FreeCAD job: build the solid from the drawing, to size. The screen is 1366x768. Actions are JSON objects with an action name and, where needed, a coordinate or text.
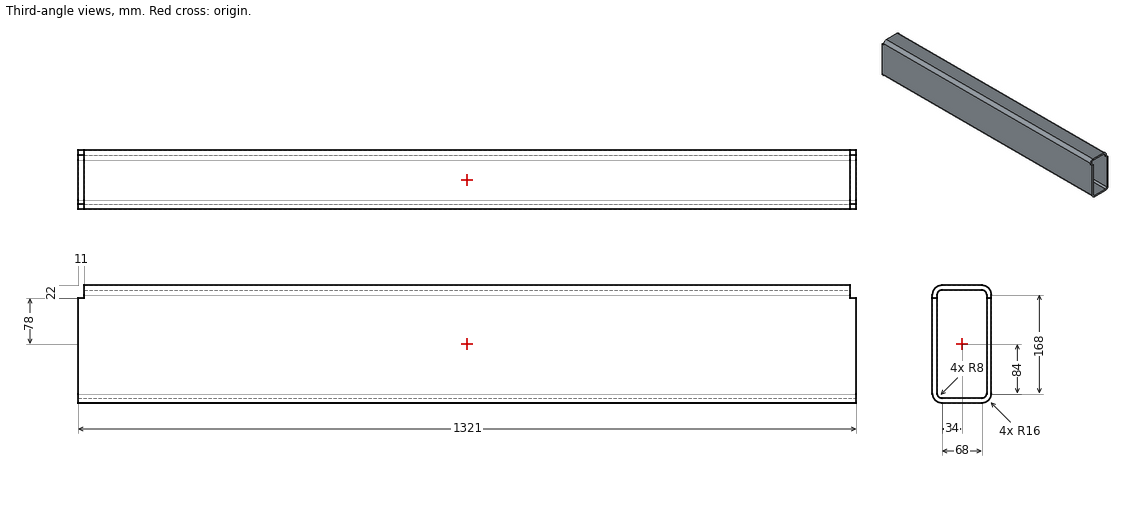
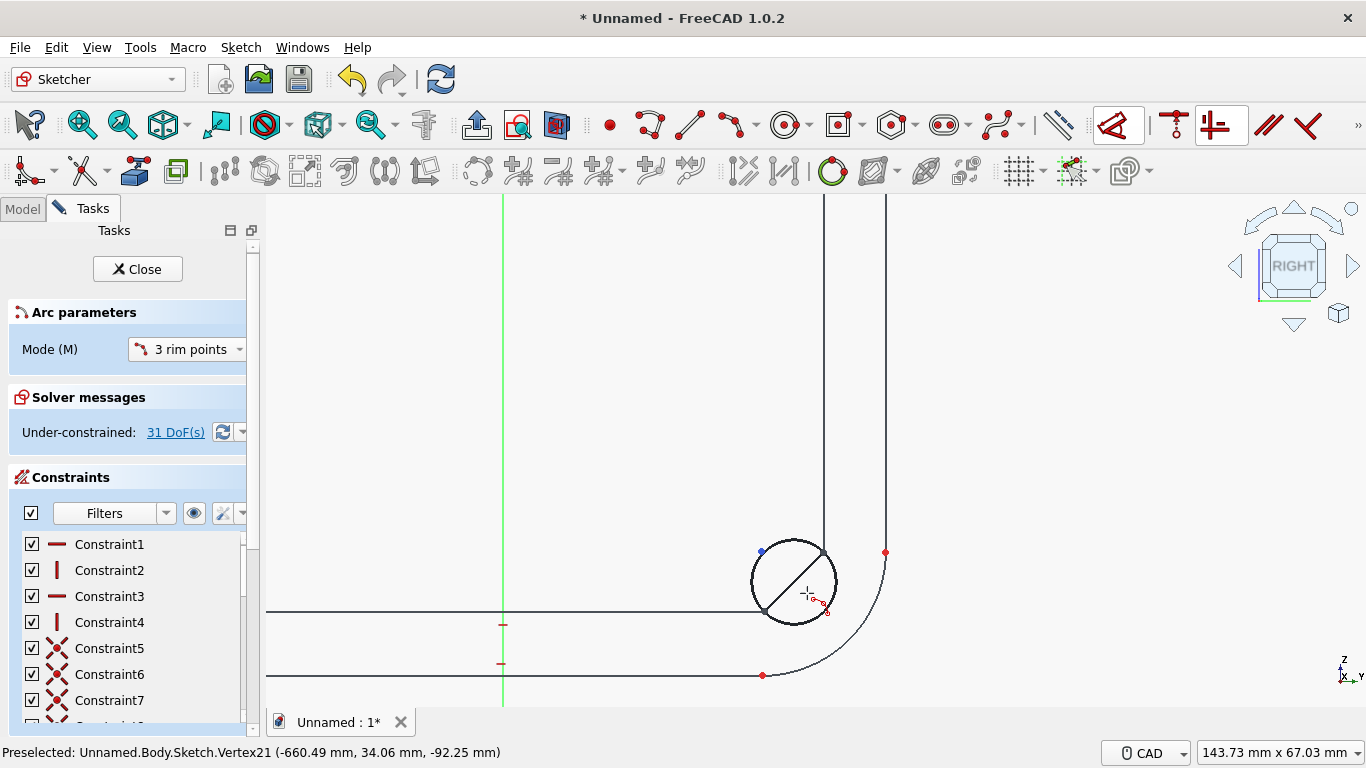
{"action": "left_click", "coordinate": [807, 592]}
{"action": "key", "text": "Escape"}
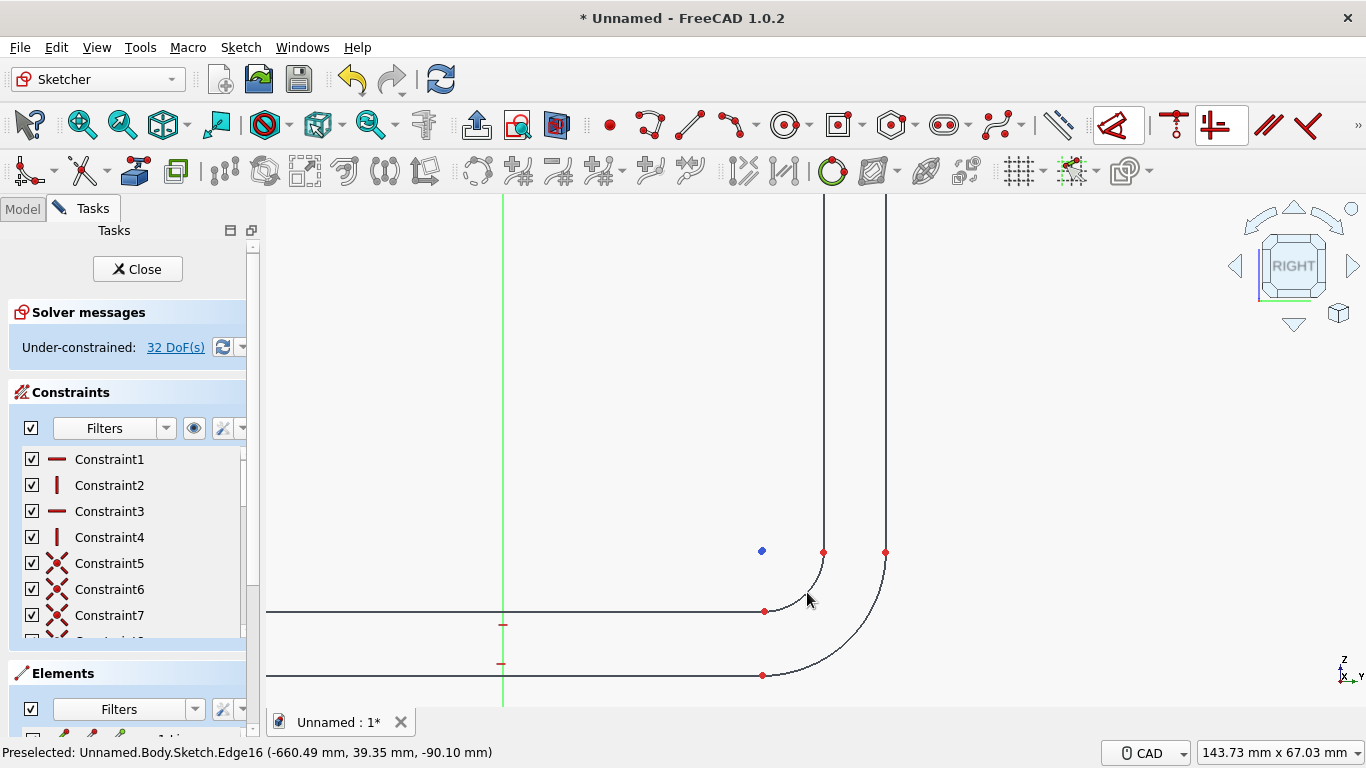
{"action": "scroll", "coordinate": [809, 588], "scroll_direction": "down", "scroll_amount": 8}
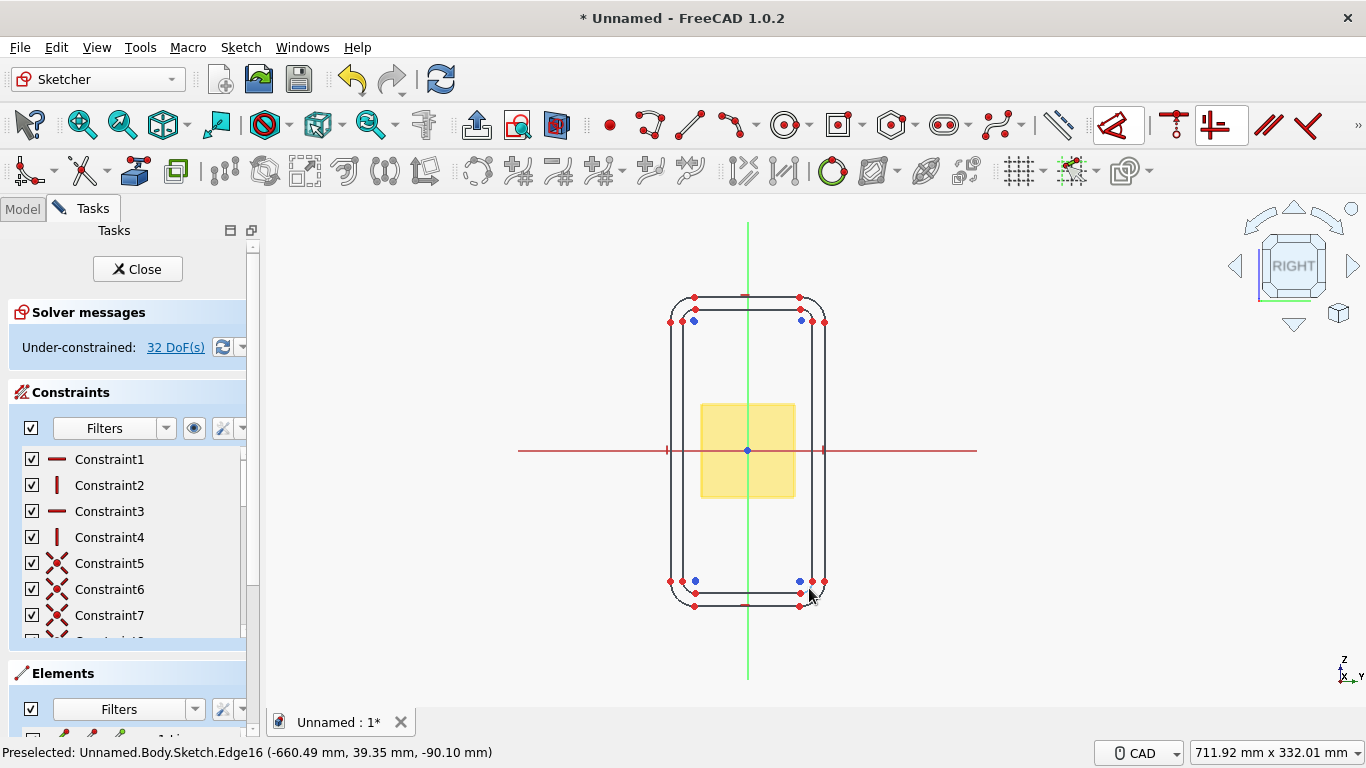
{"action": "left_click", "coordinate": [726, 606]}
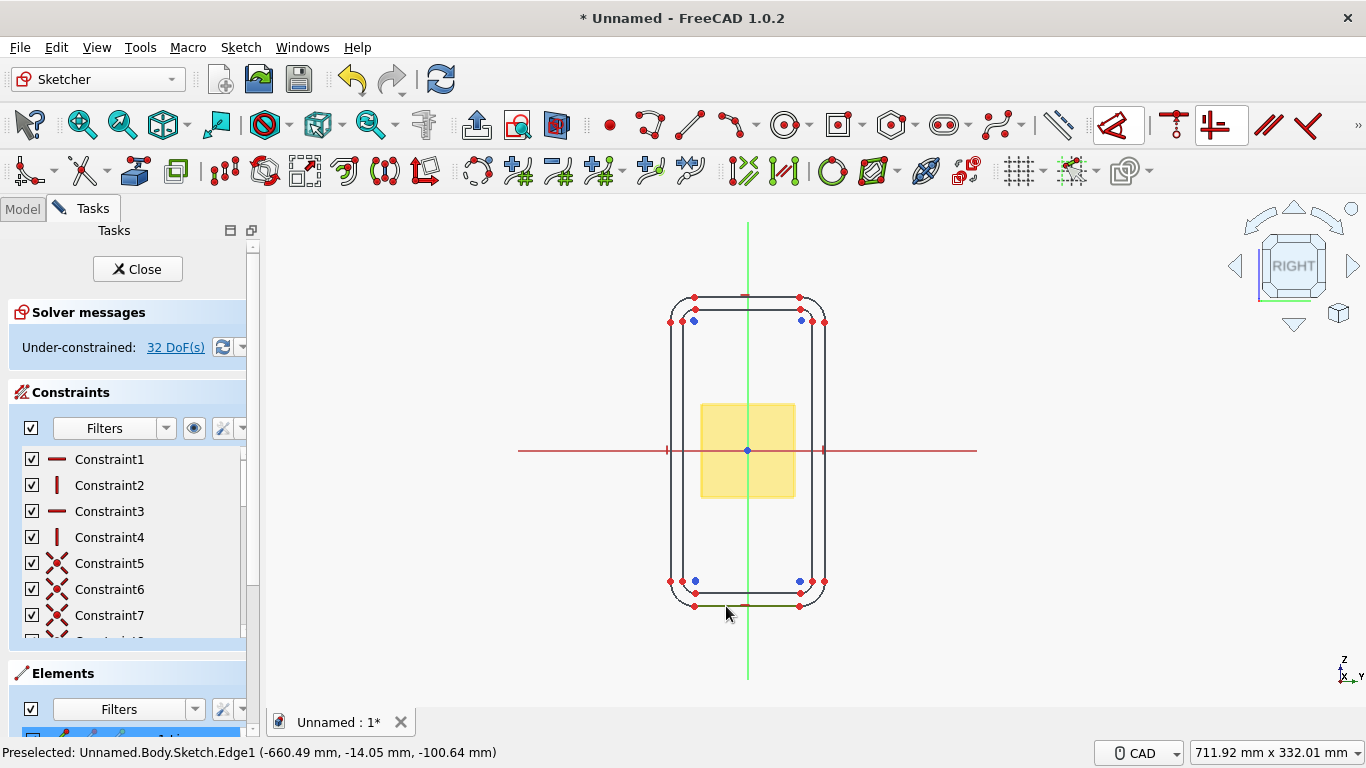
{"action": "left_click", "coordinate": [811, 604]}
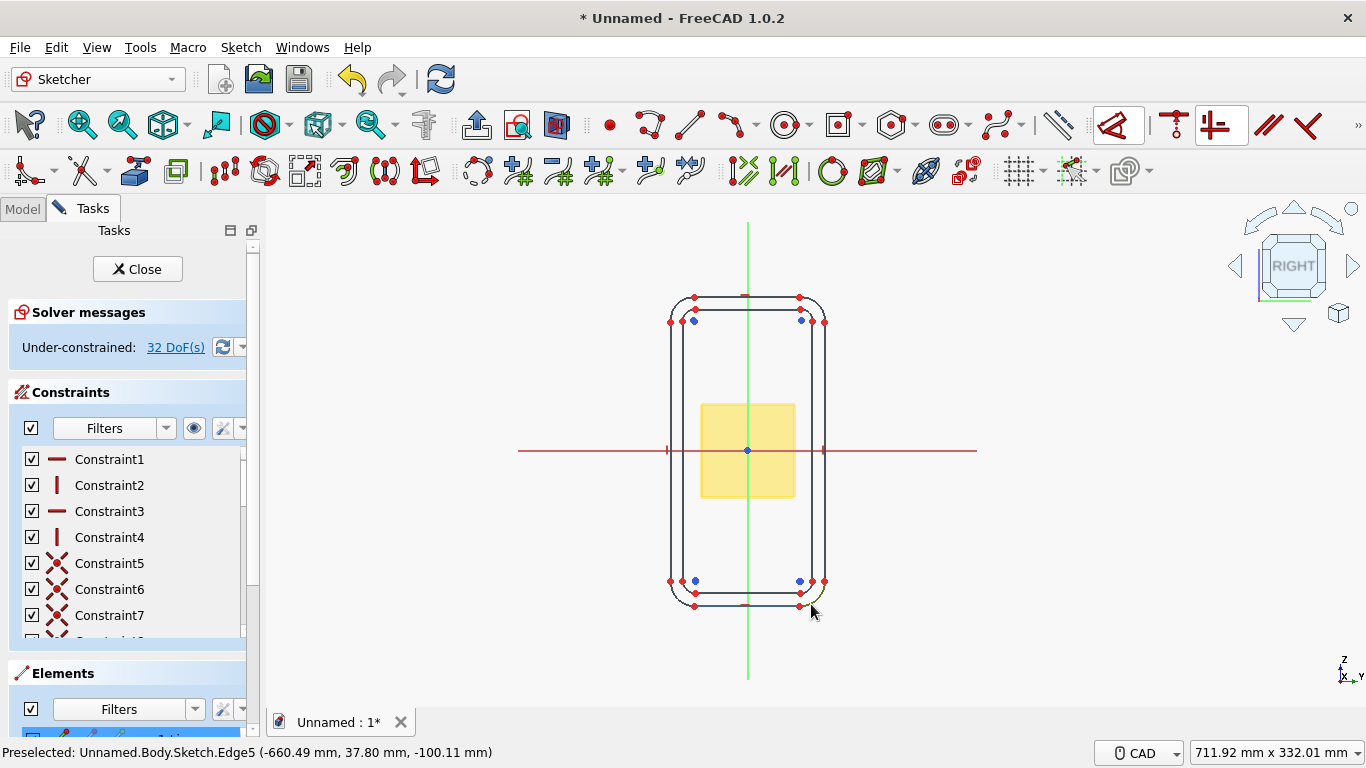
{"action": "key", "text": "t"}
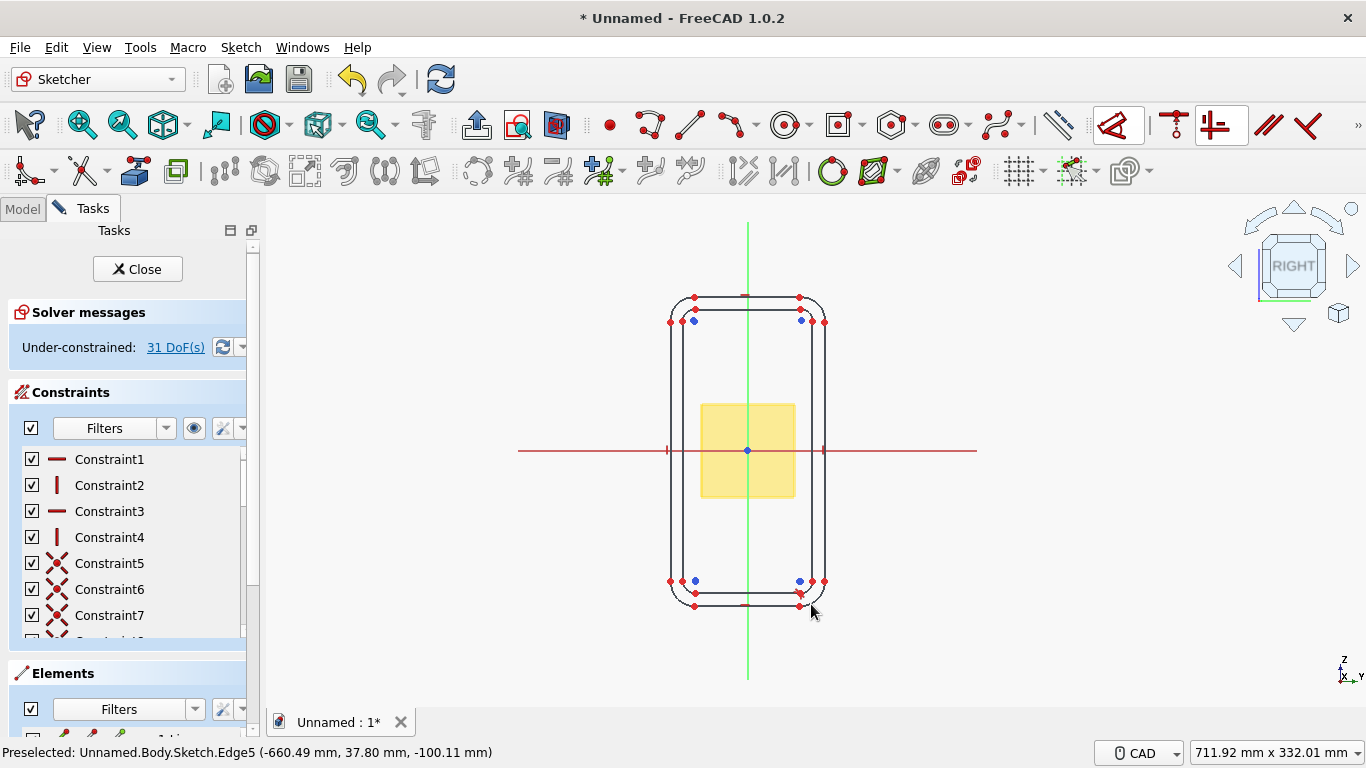
{"action": "left_click", "coordinate": [726, 606]}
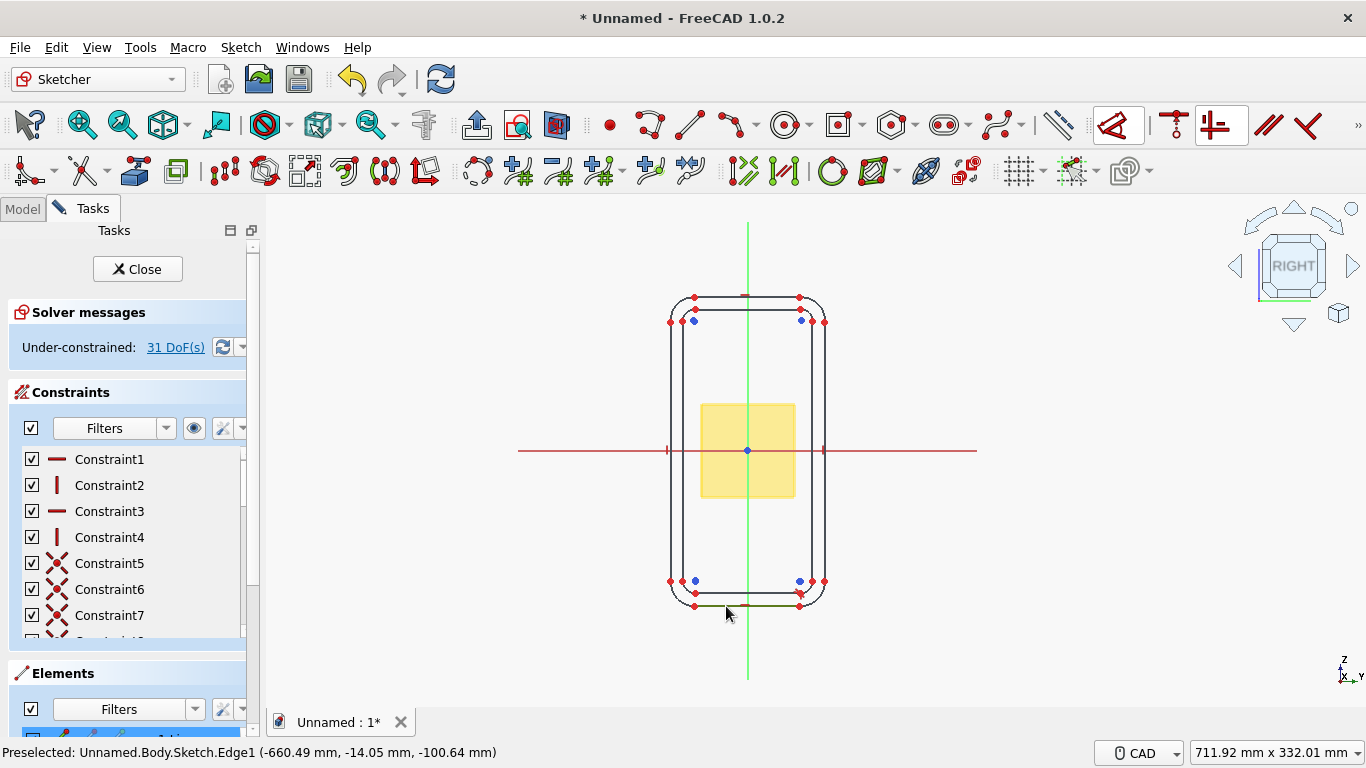
{"action": "left_click", "coordinate": [673, 593]}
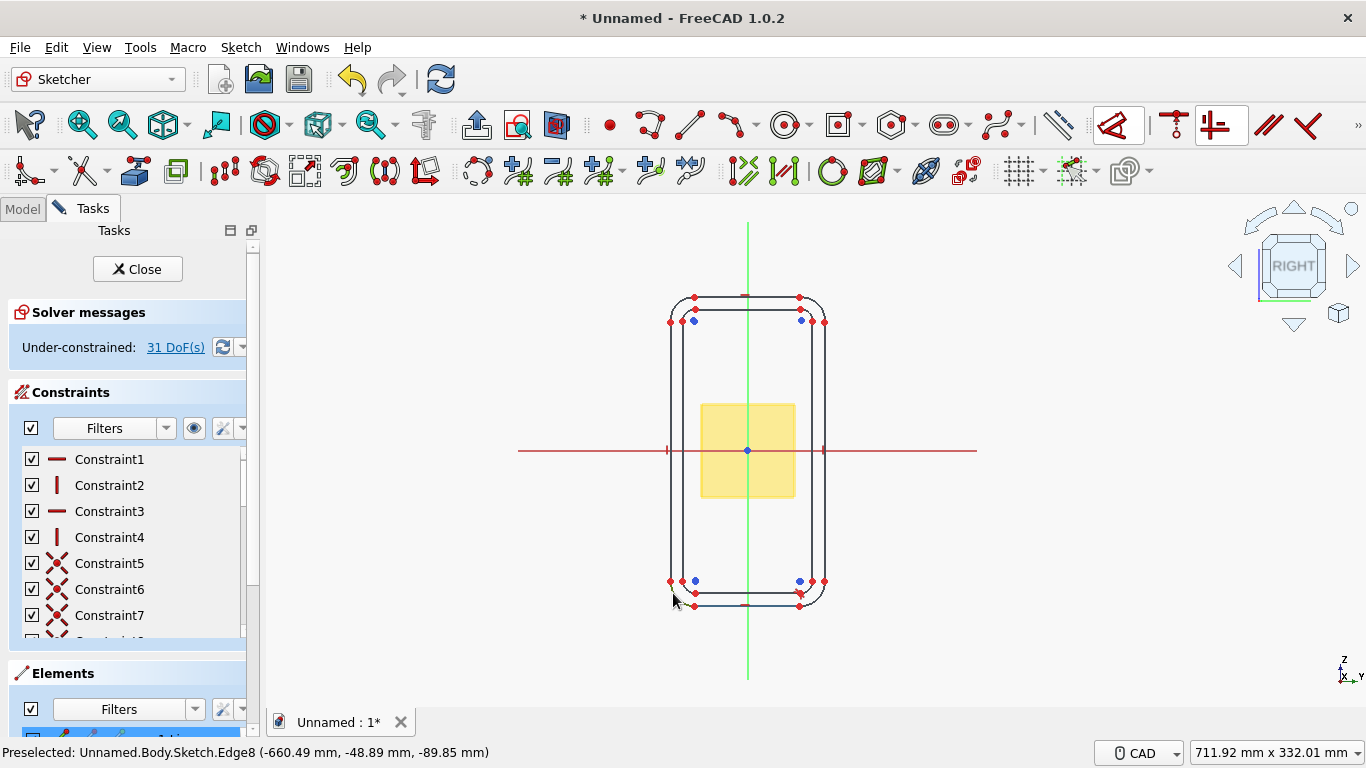
{"action": "key", "text": "t"}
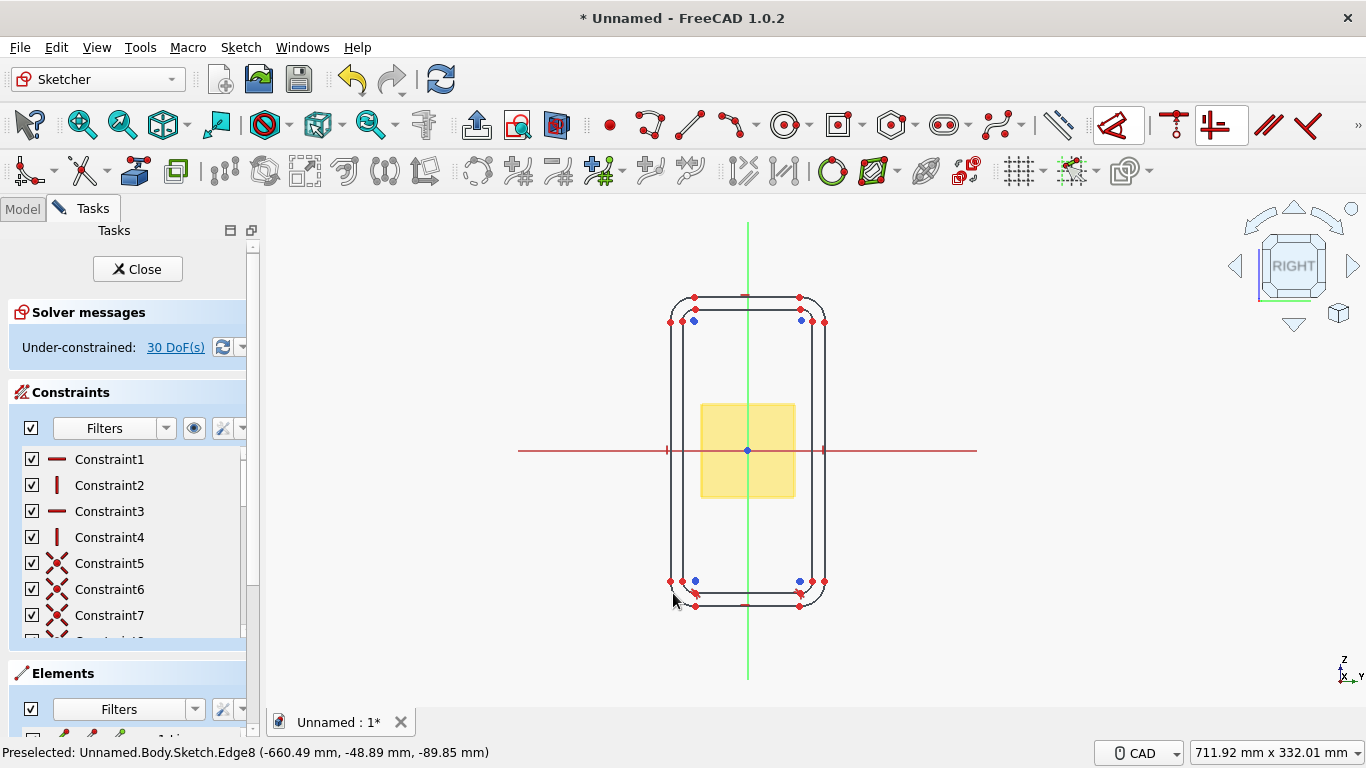
{"action": "left_click", "coordinate": [825, 504]}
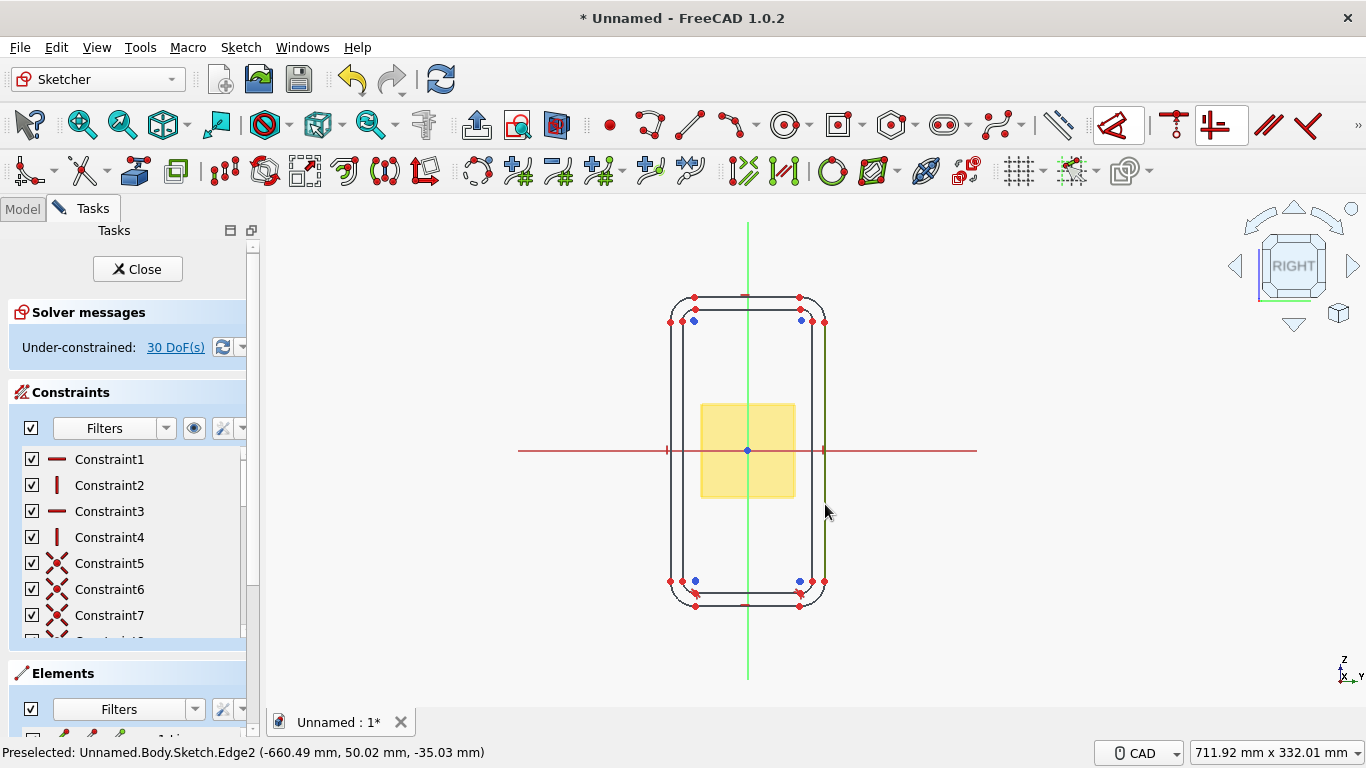
{"action": "left_click", "coordinate": [811, 604]}